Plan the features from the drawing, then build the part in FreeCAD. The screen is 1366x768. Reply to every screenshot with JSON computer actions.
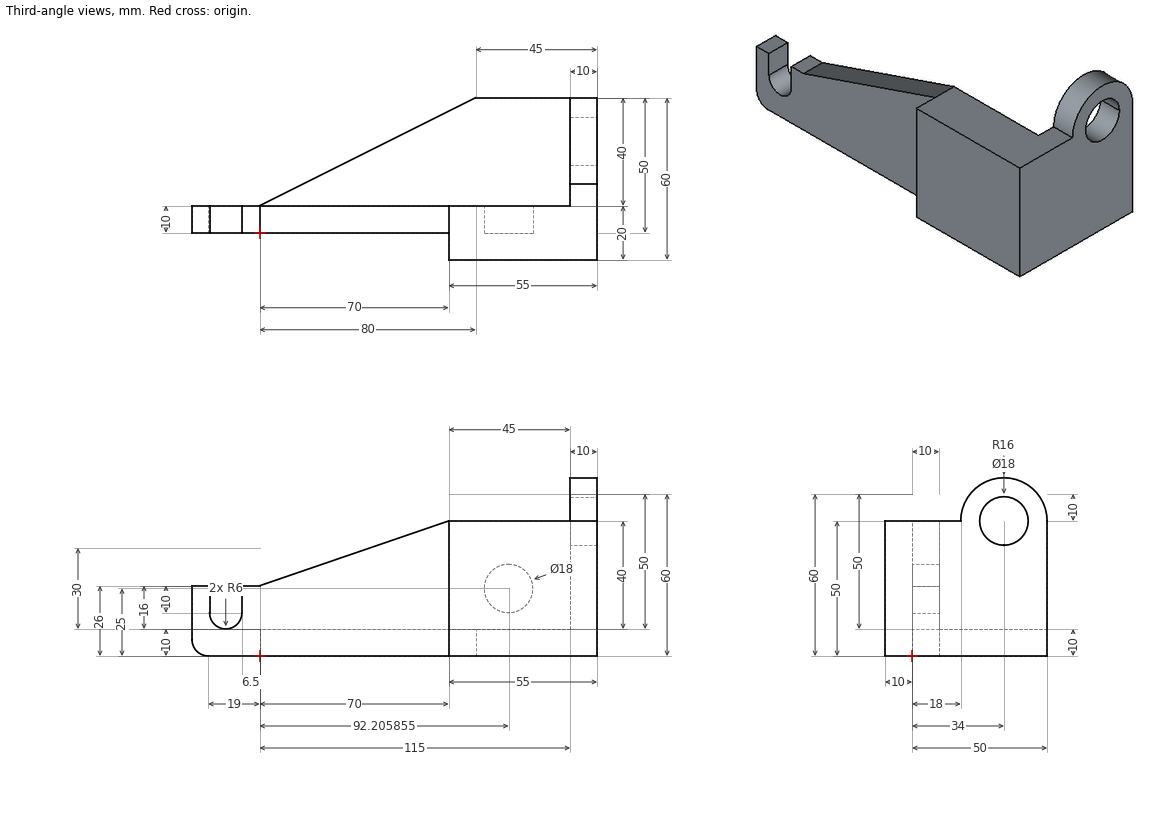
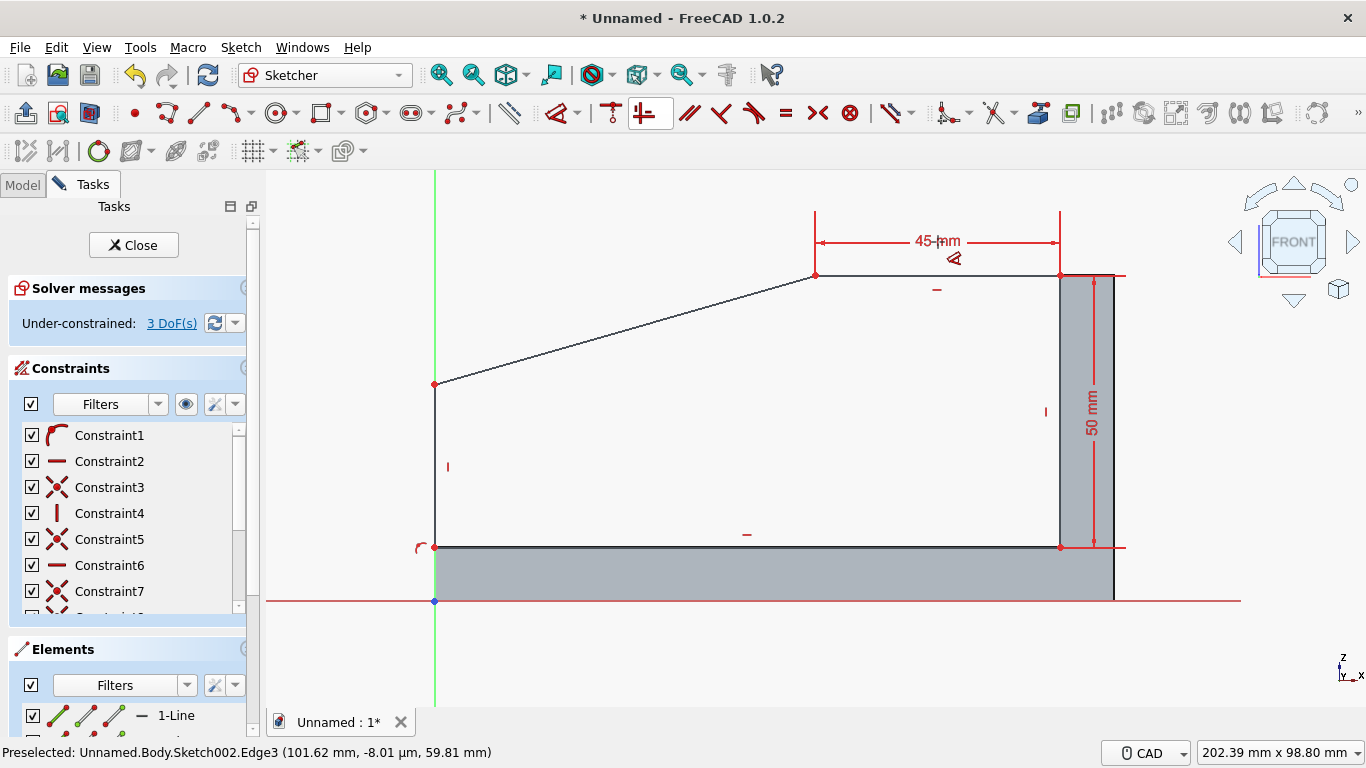
{"action": "left_click", "coordinate": [435, 434]}
{"action": "left_click", "coordinate": [401, 466]}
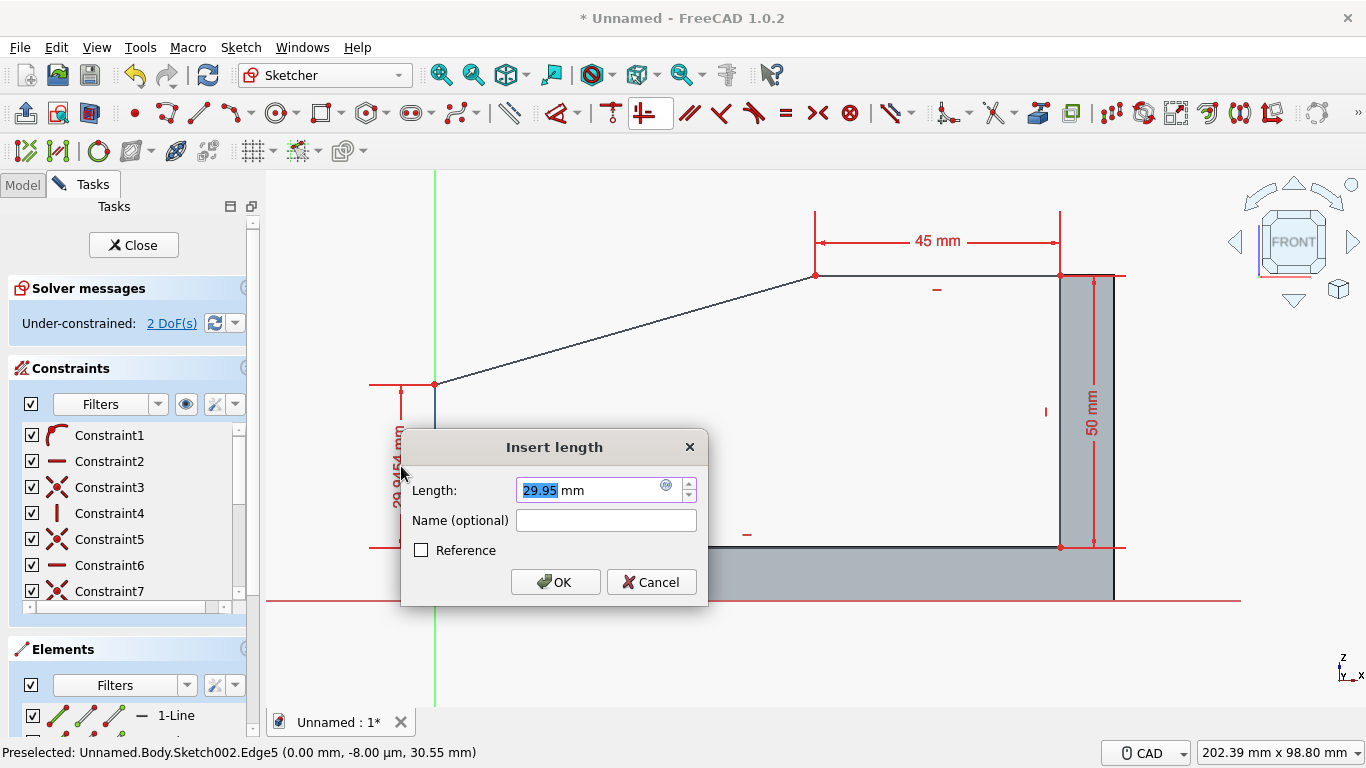
{"action": "type", "text": "30"}
{"action": "key", "text": "Return"}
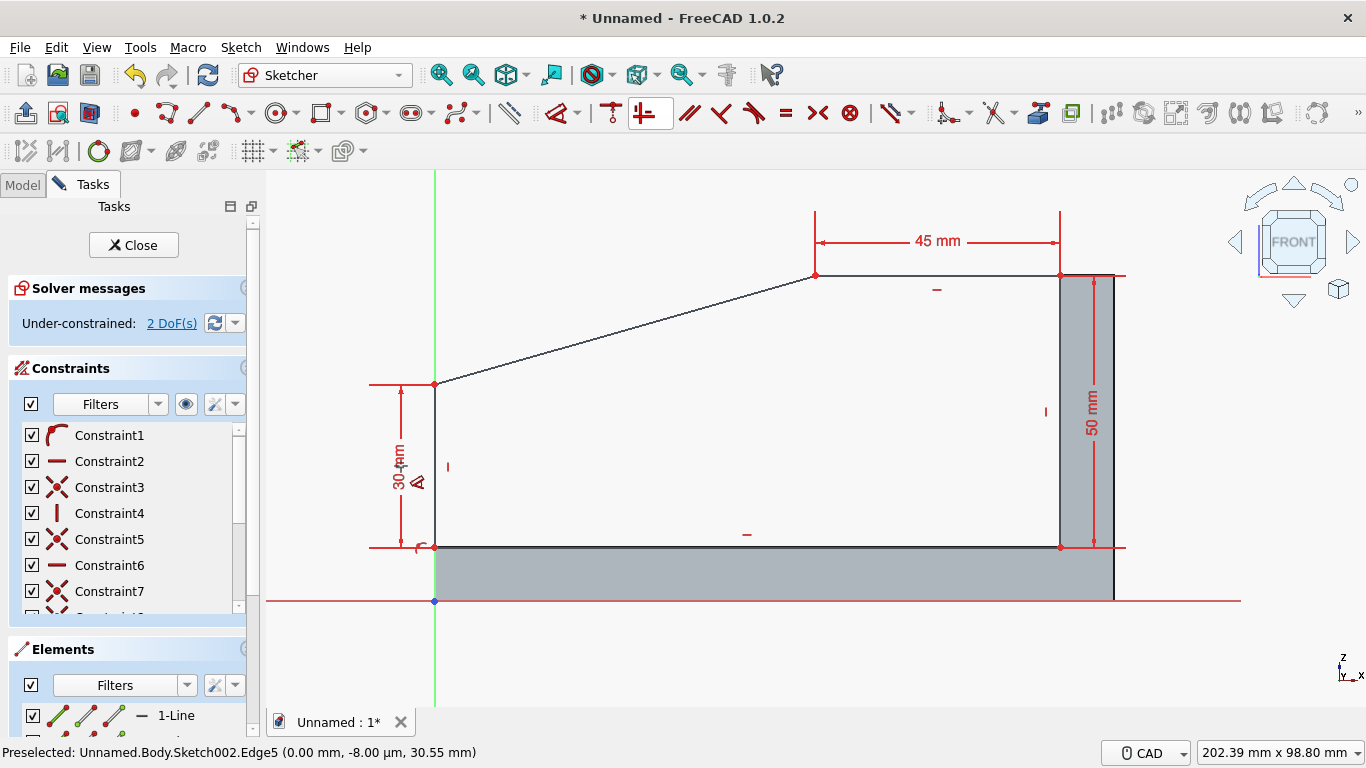
{"action": "left_click", "coordinate": [622, 548]}
{"action": "left_click", "coordinate": [747, 582]}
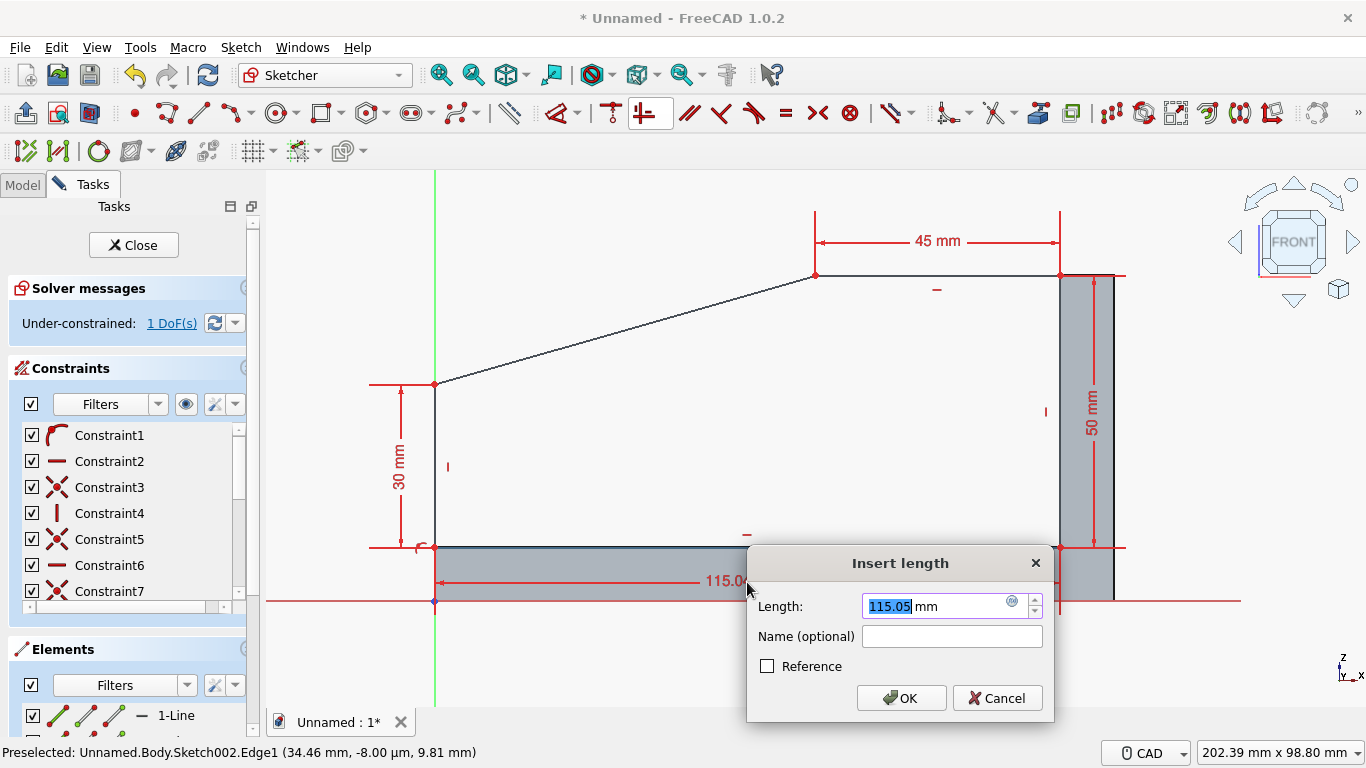
{"action": "type", "text": "115"}
{"action": "key", "text": "Return"}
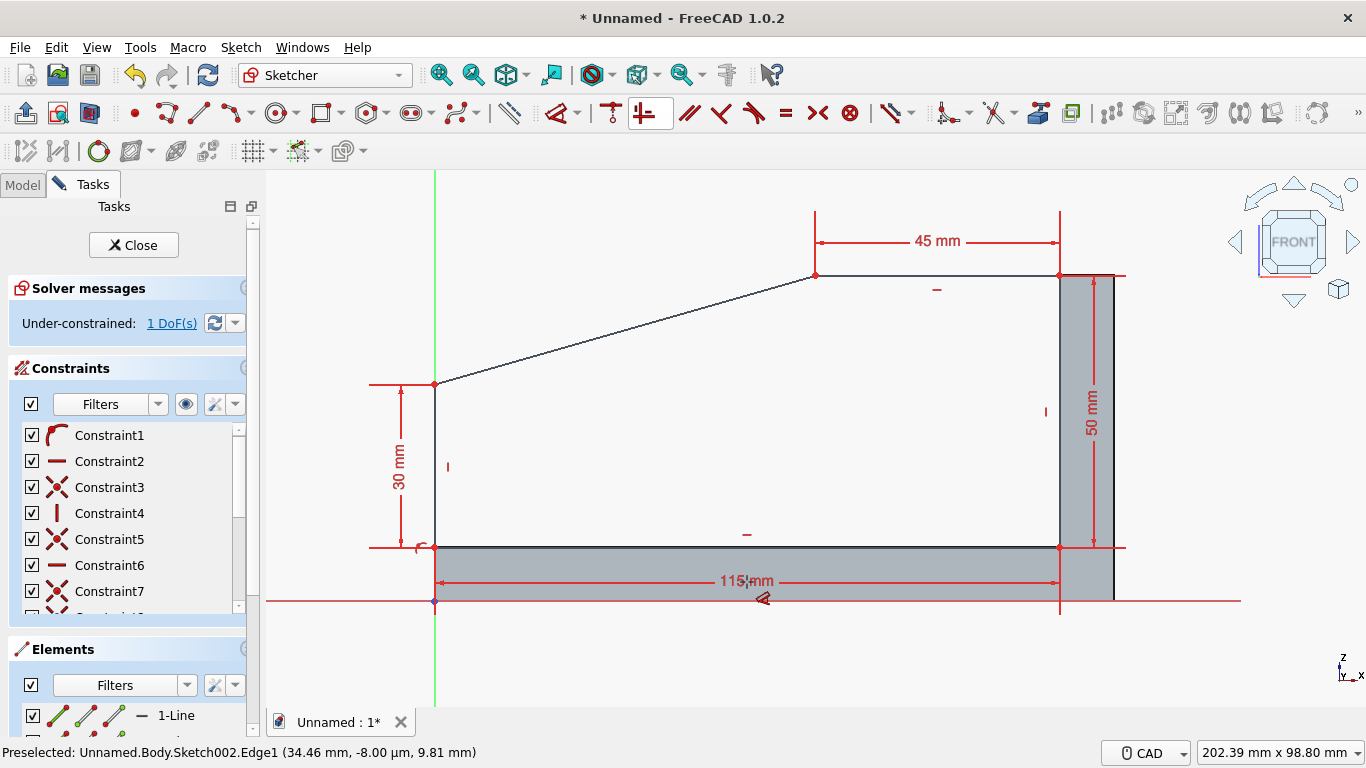
{"action": "left_click", "coordinate": [435, 548]}
{"action": "left_click", "coordinate": [401, 574]}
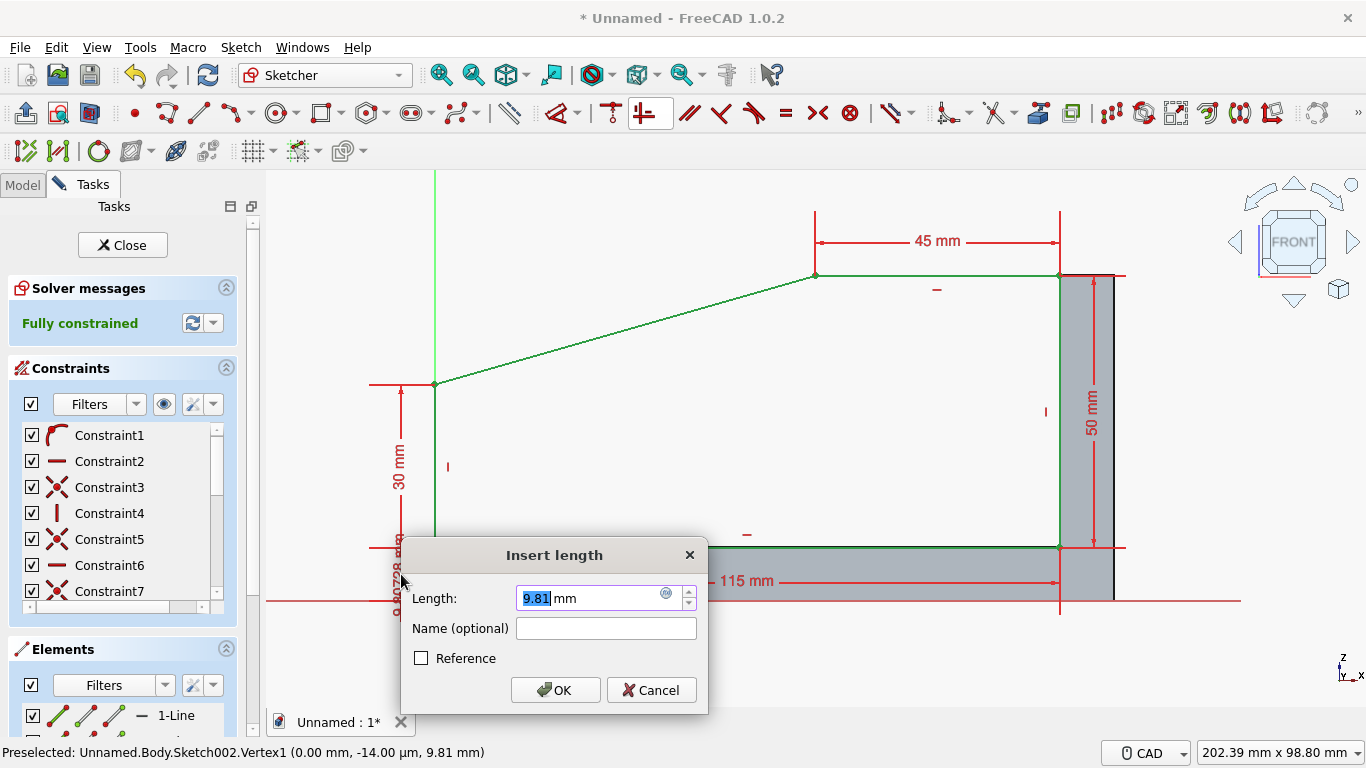
{"action": "type", "text": "10"}
{"action": "key", "text": "Return"}
{"action": "key", "text": "Escape"}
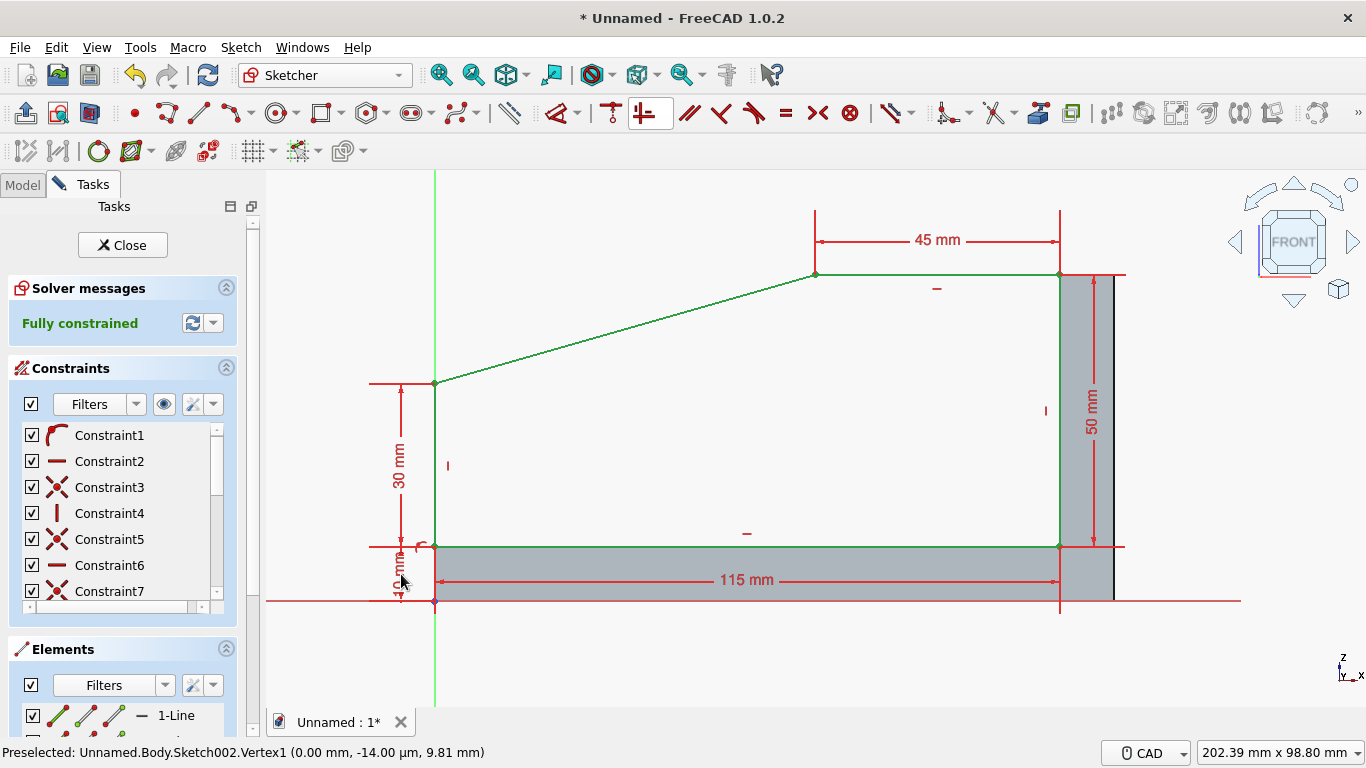
{"action": "left_click", "coordinate": [123, 245]}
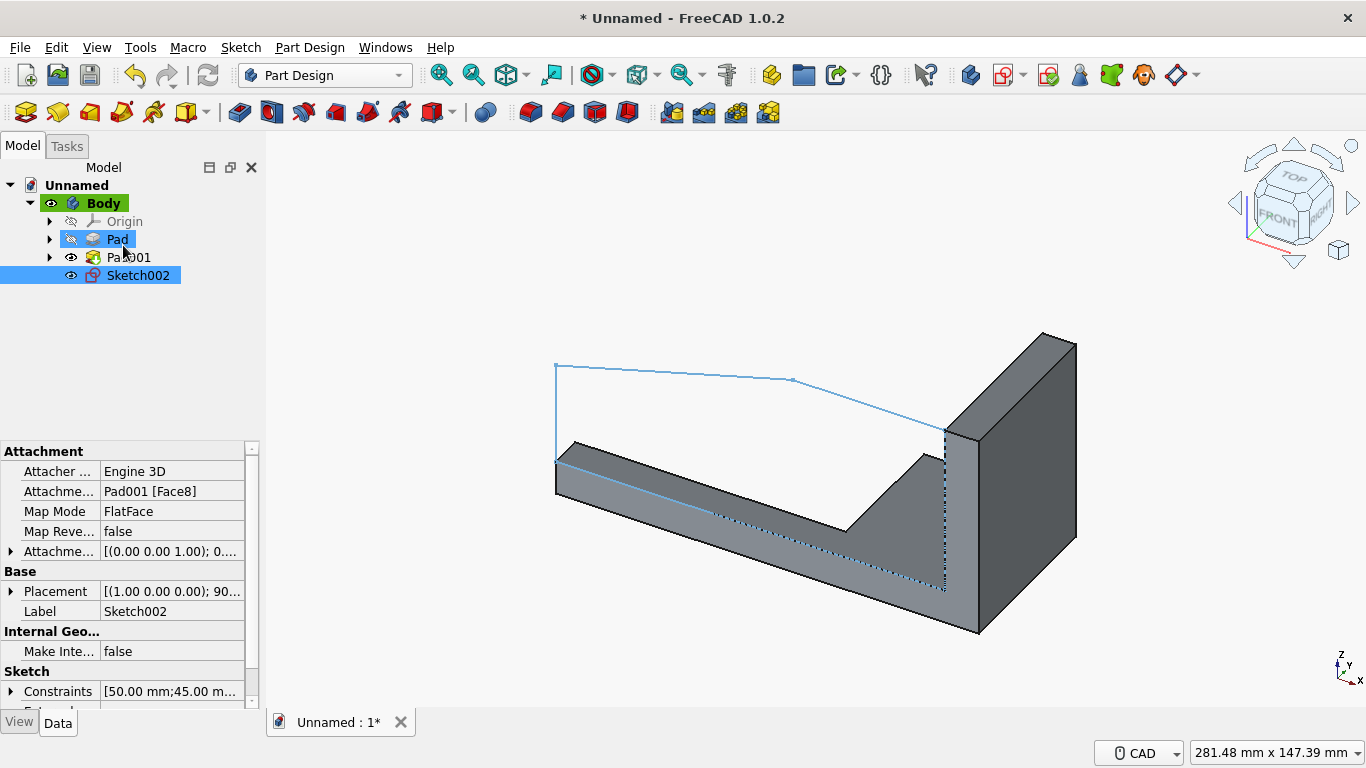
{"action": "left_click", "coordinate": [26, 112]}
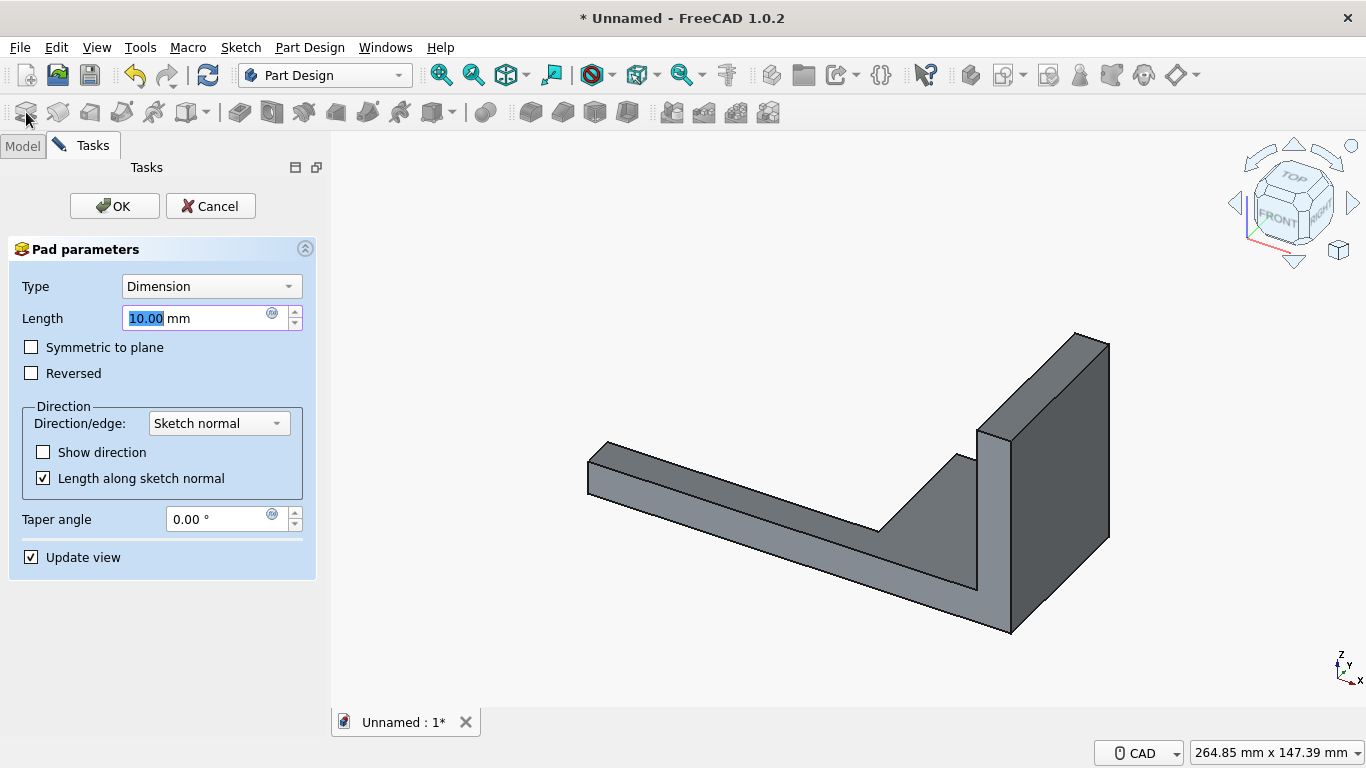
{"action": "type", "text": "10"}
{"action": "key", "text": "Tab"}